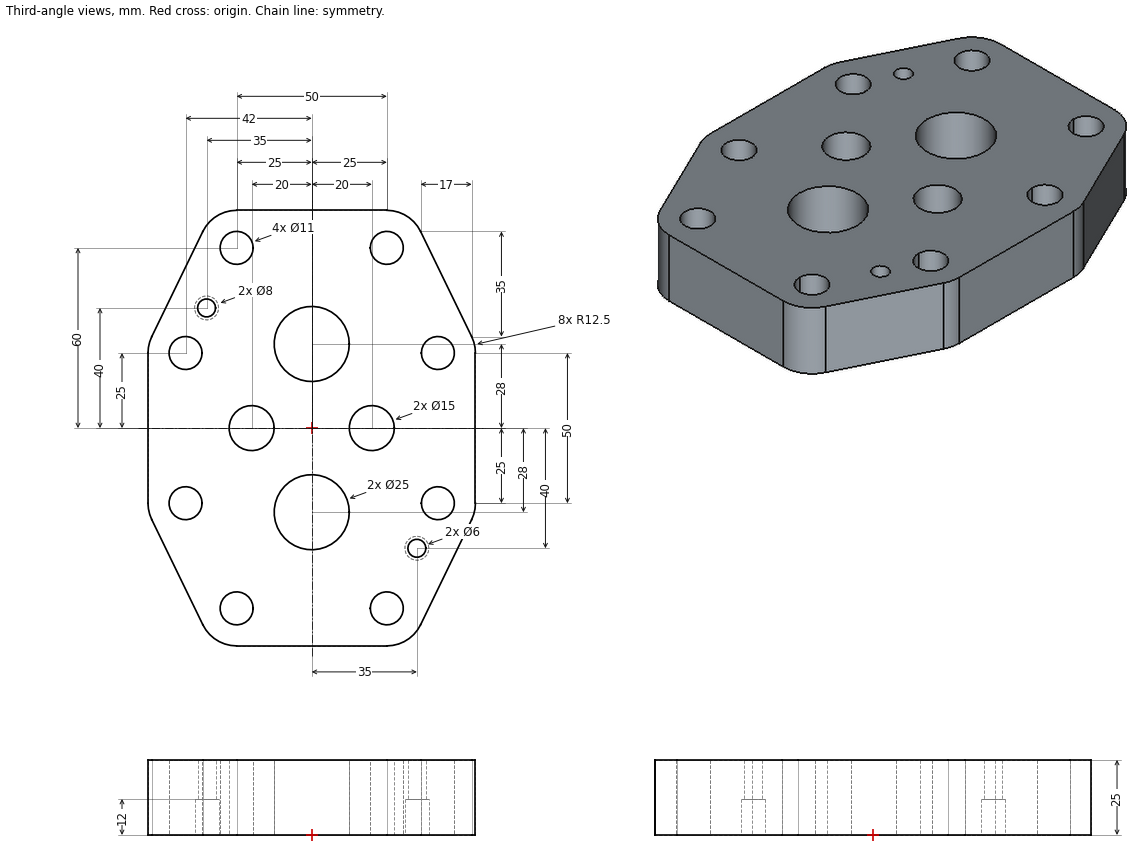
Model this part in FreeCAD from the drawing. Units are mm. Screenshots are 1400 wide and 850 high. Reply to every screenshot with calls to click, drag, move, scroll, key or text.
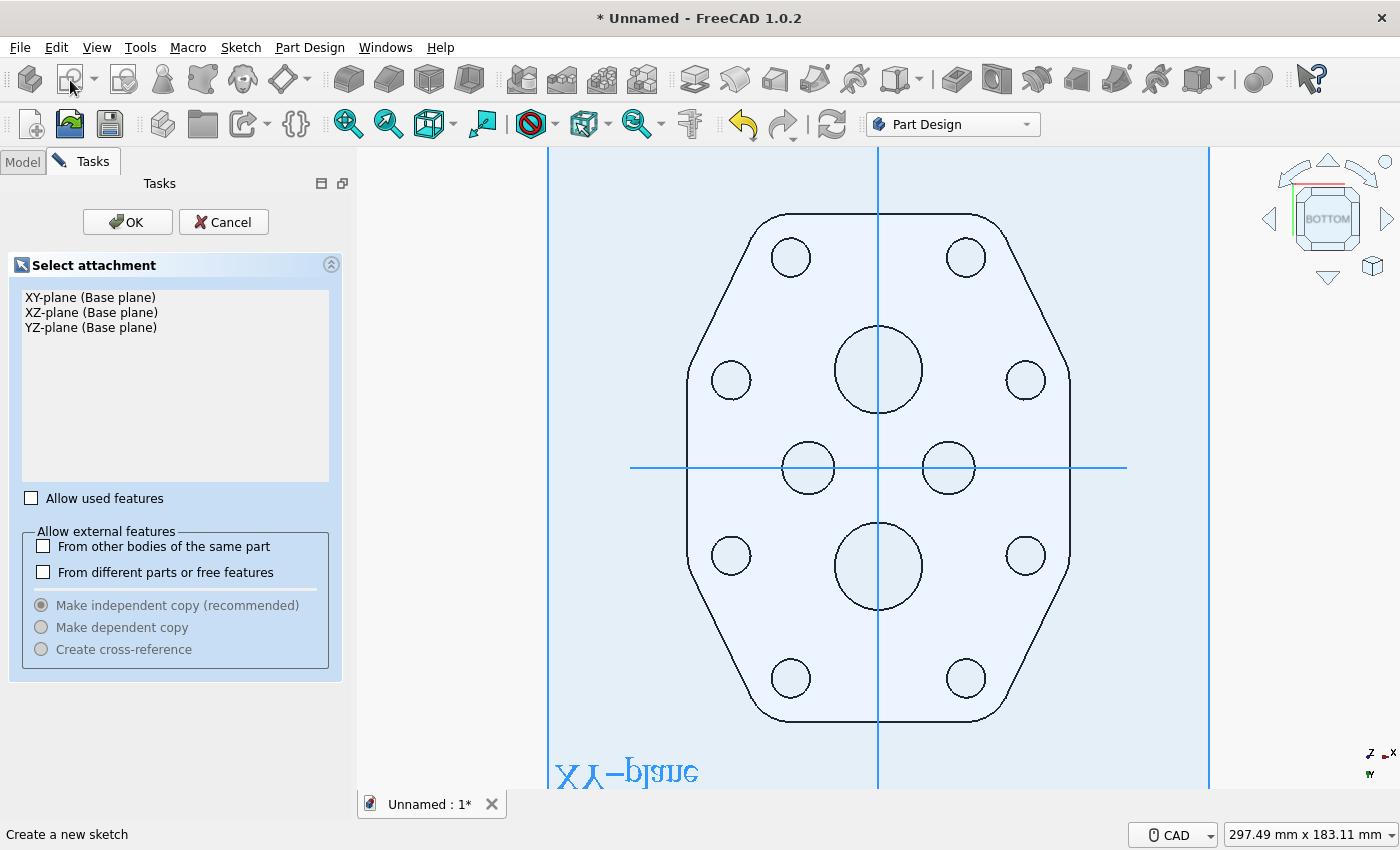
click(82, 298)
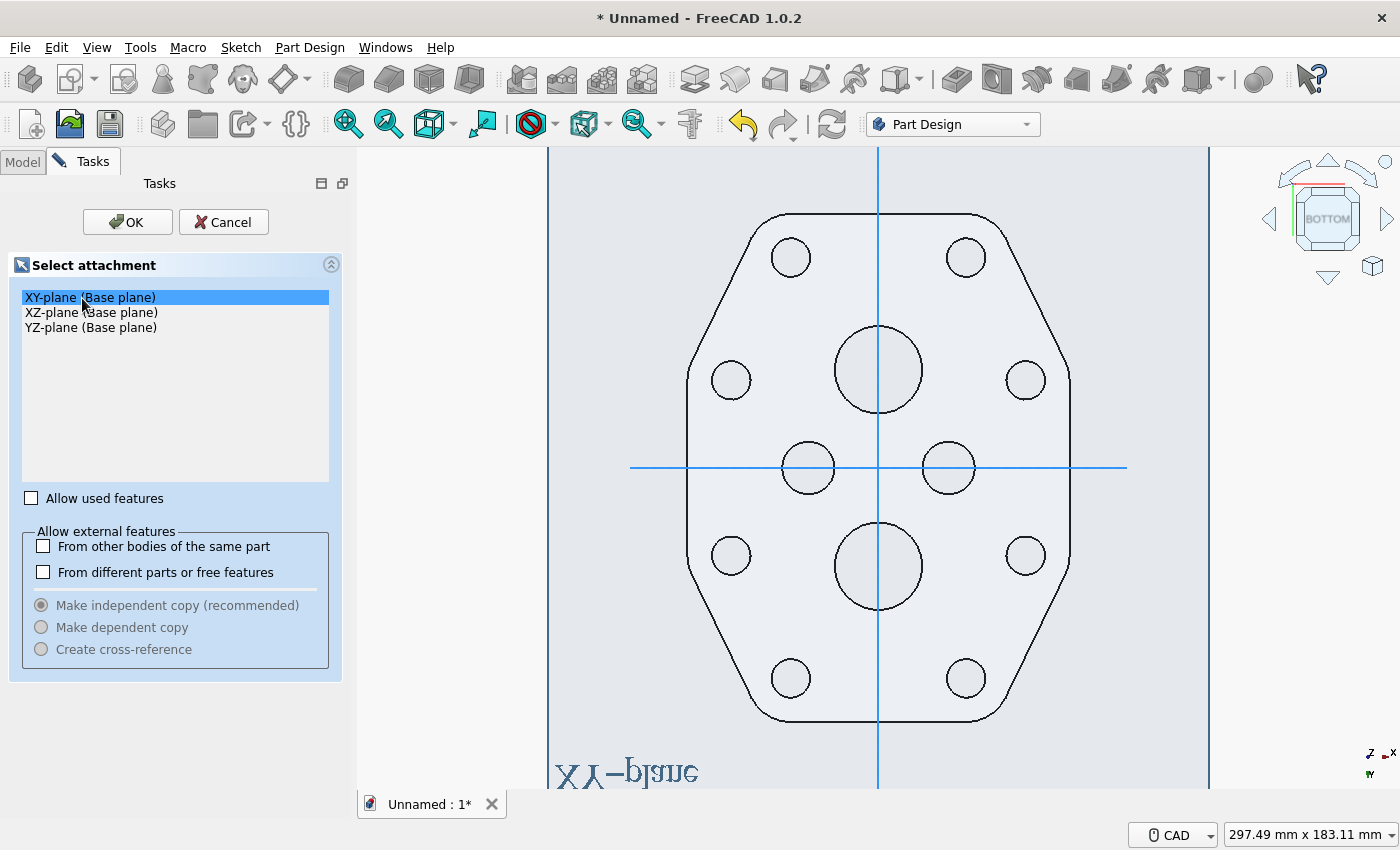
click(128, 222)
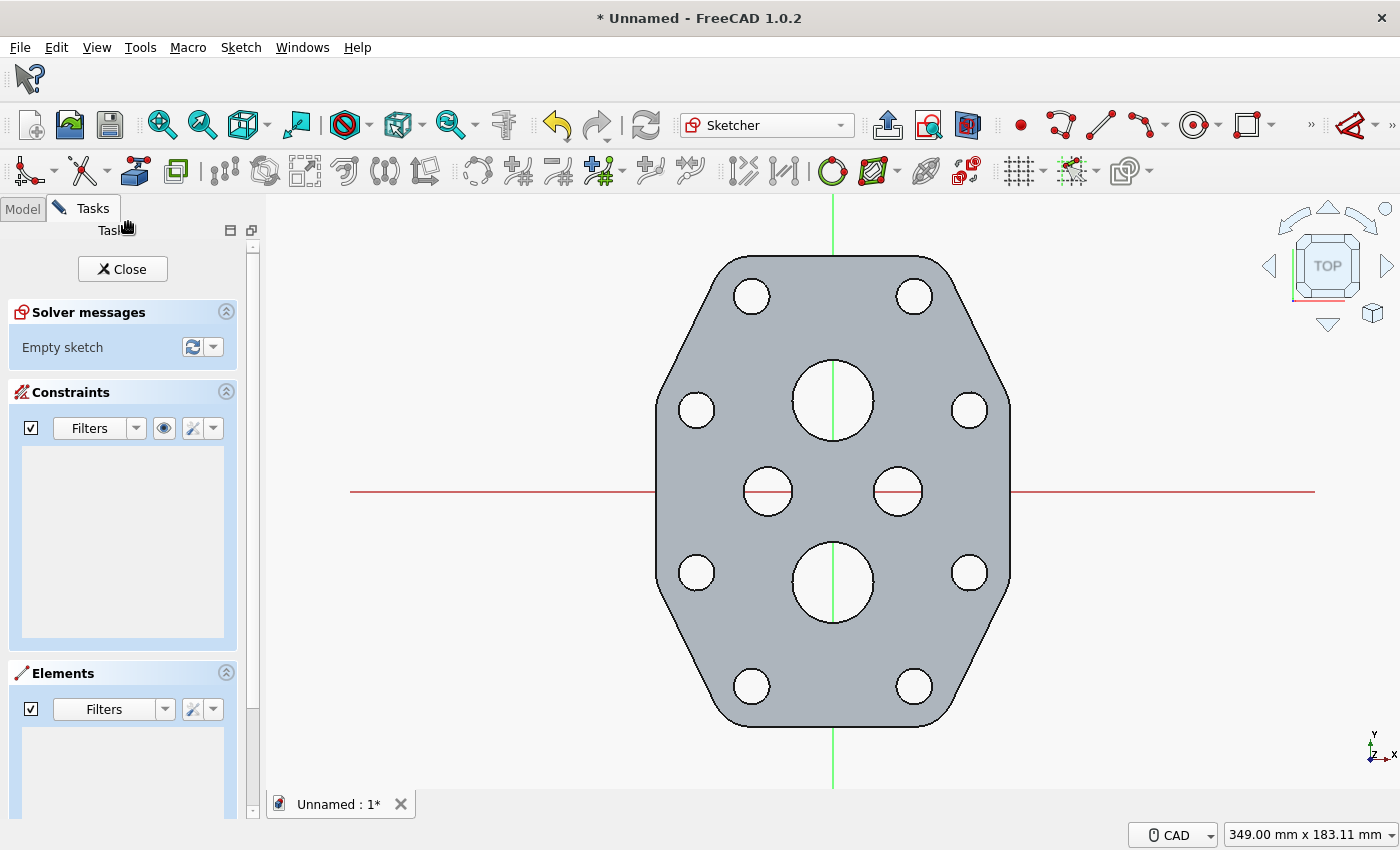
key(q)
key(s)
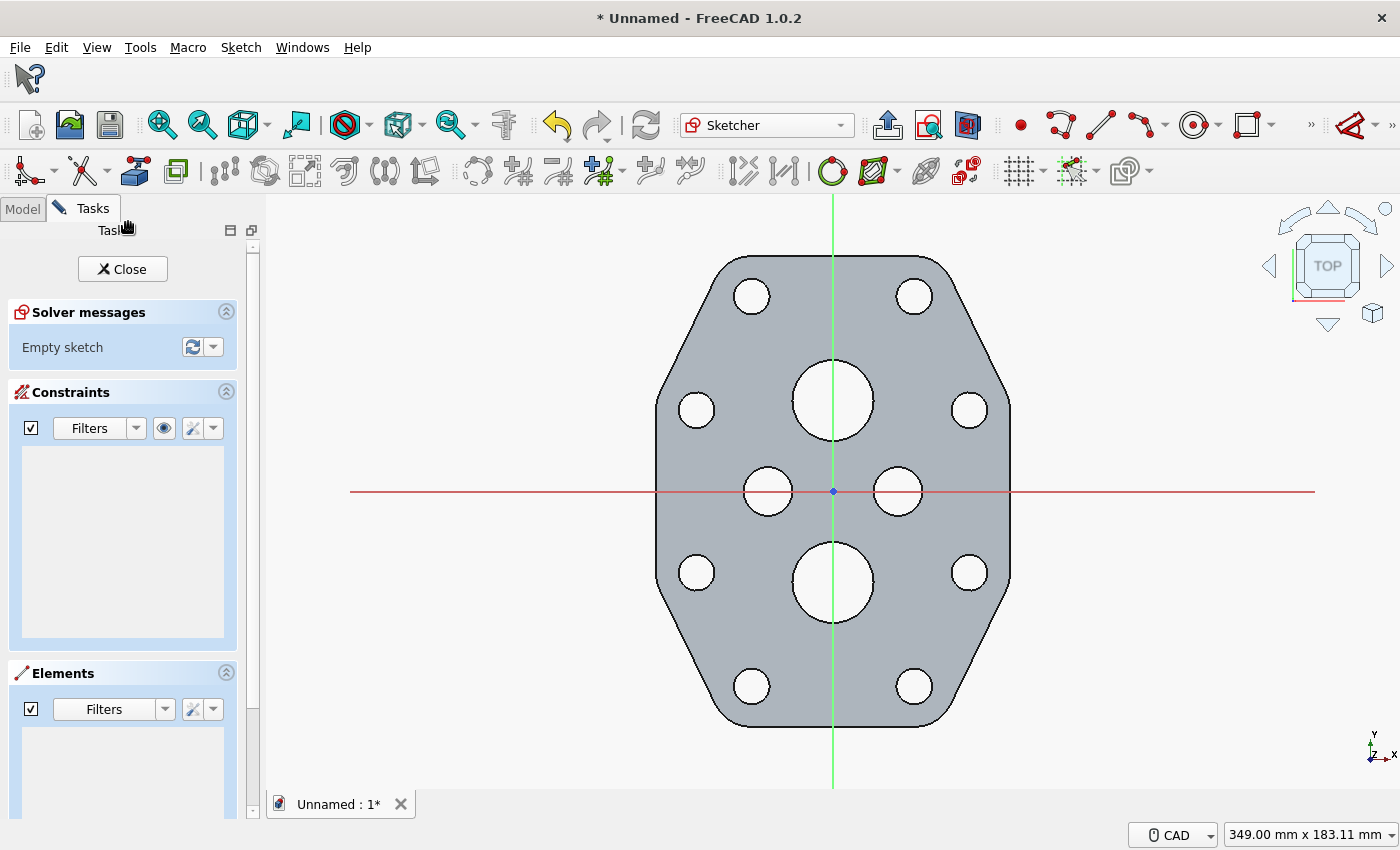
scroll(972, 491, up, 2)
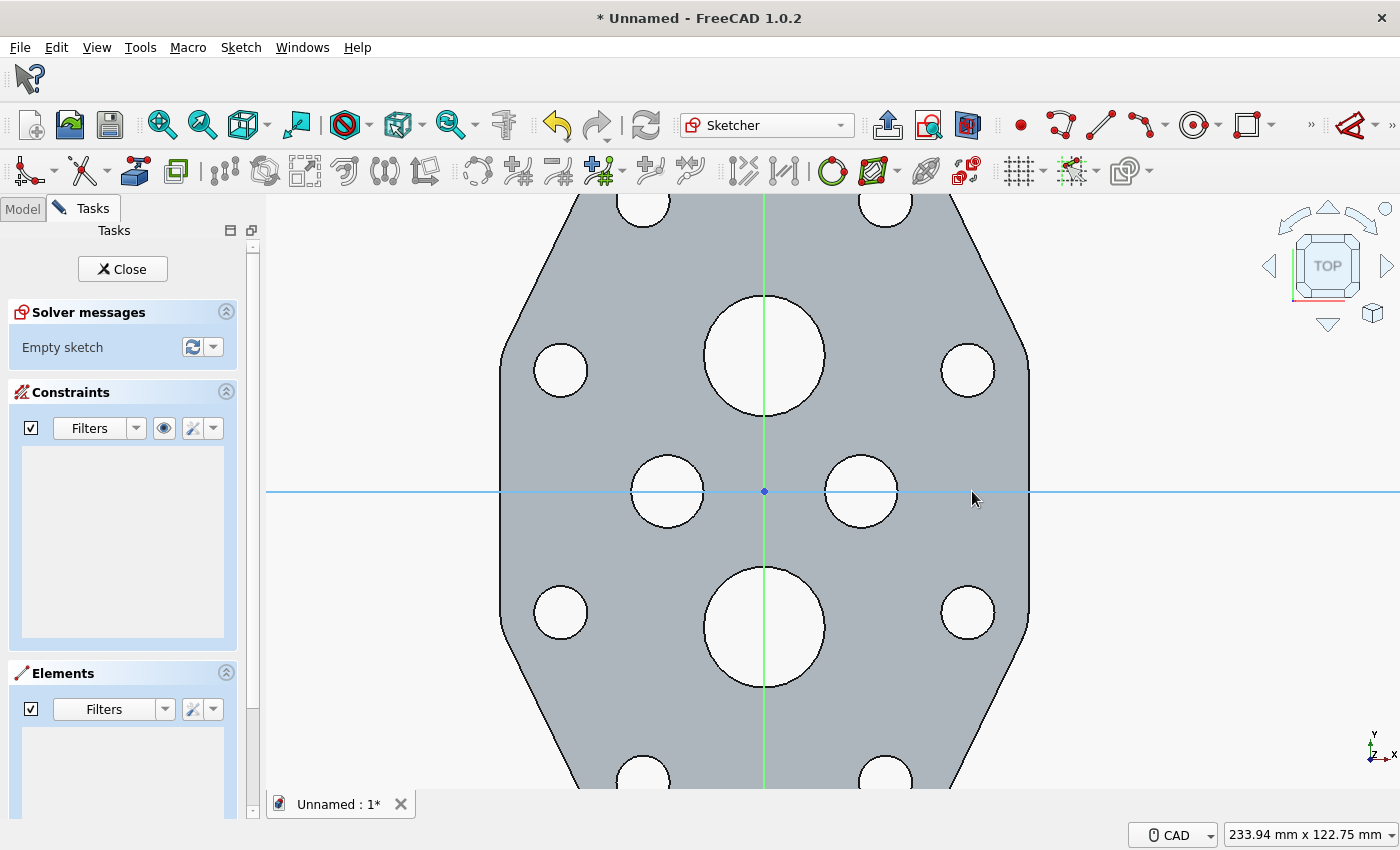
click(1194, 126)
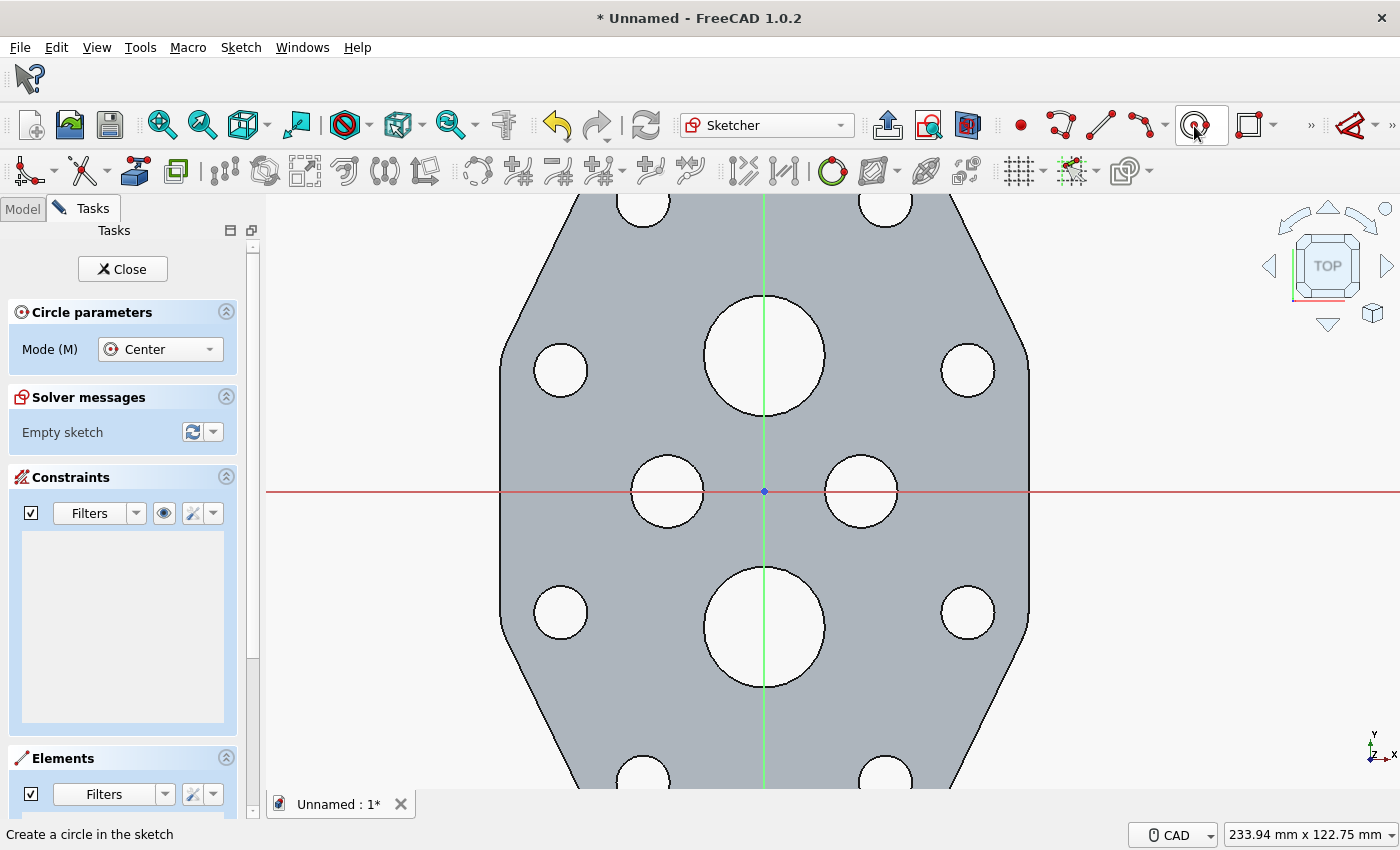
scroll(934, 685, up, 3)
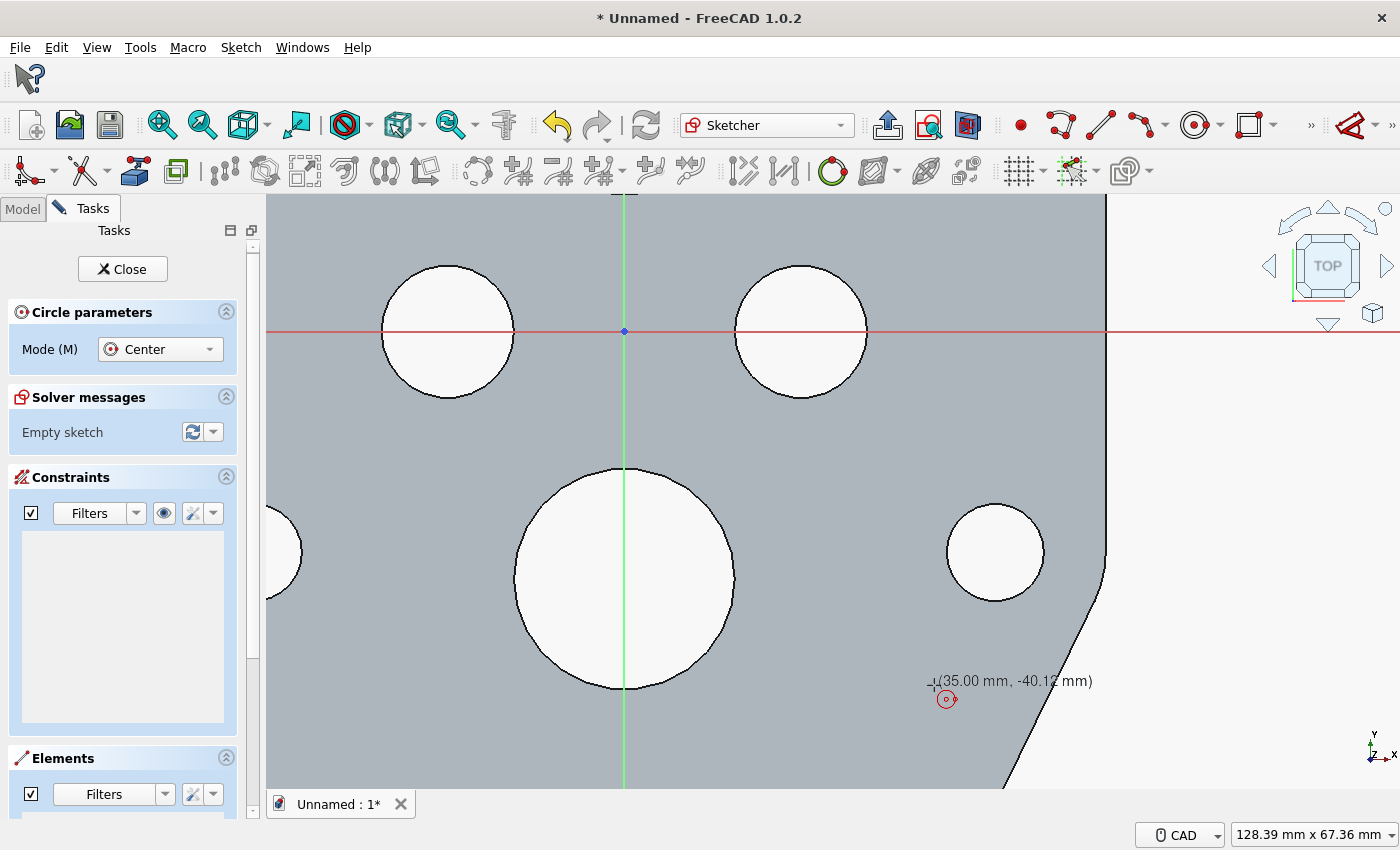
click(933, 685)
click(952, 666)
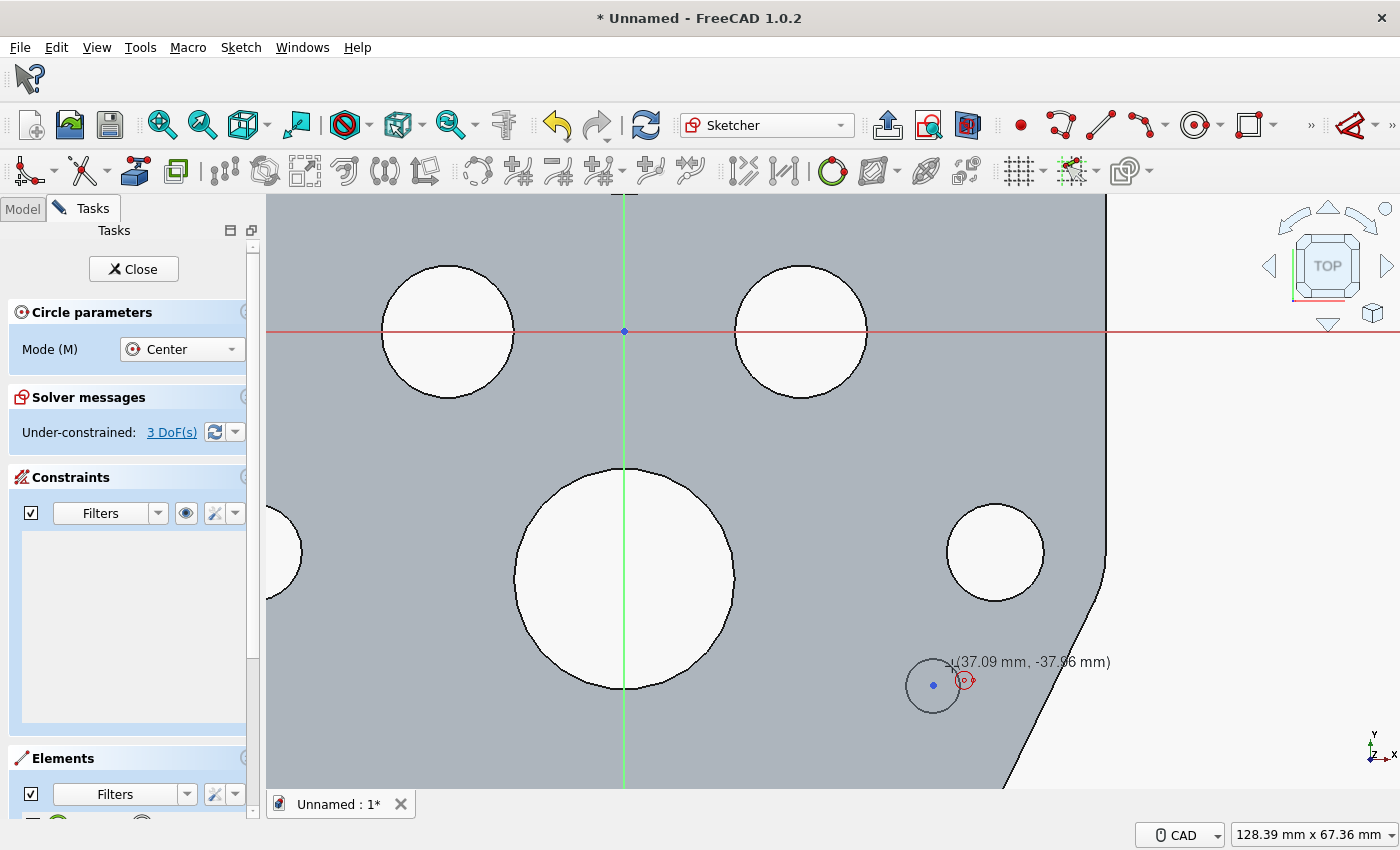
scroll(935, 686, down, 3)